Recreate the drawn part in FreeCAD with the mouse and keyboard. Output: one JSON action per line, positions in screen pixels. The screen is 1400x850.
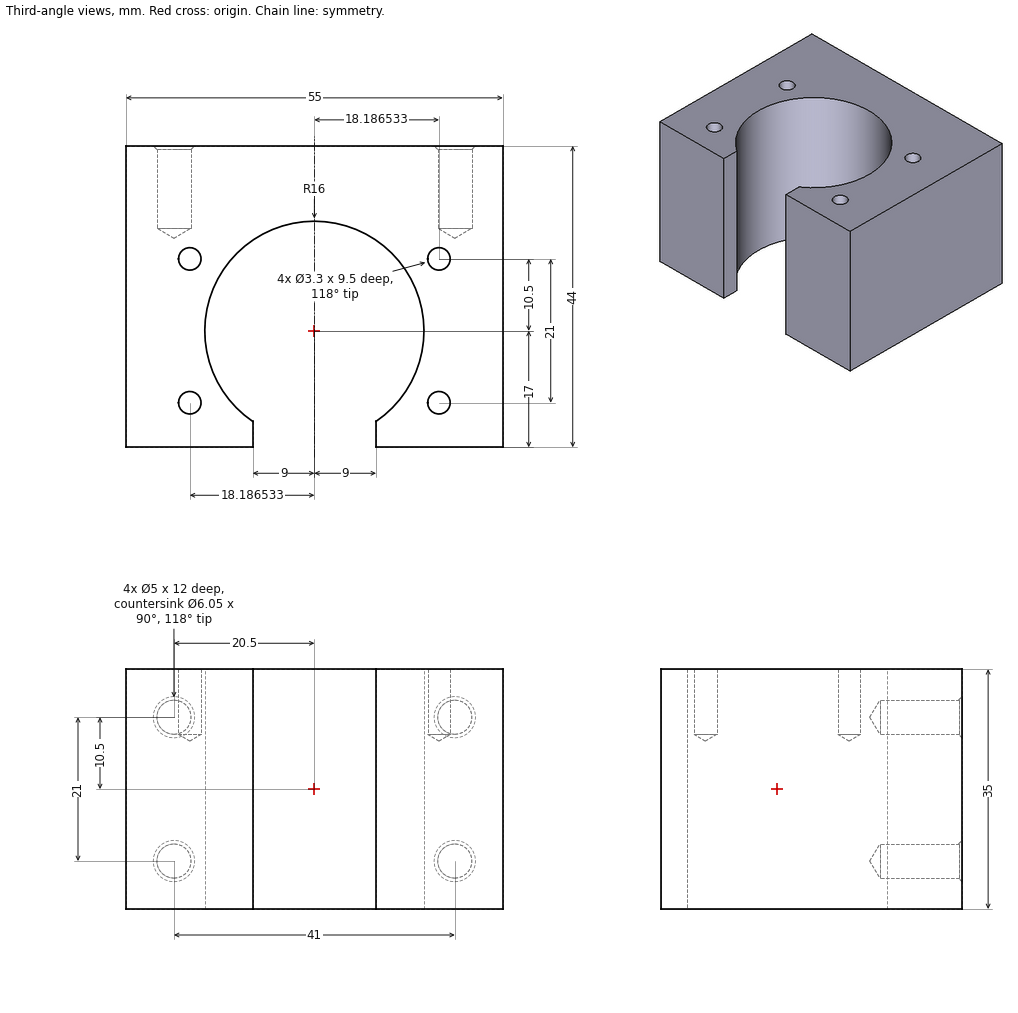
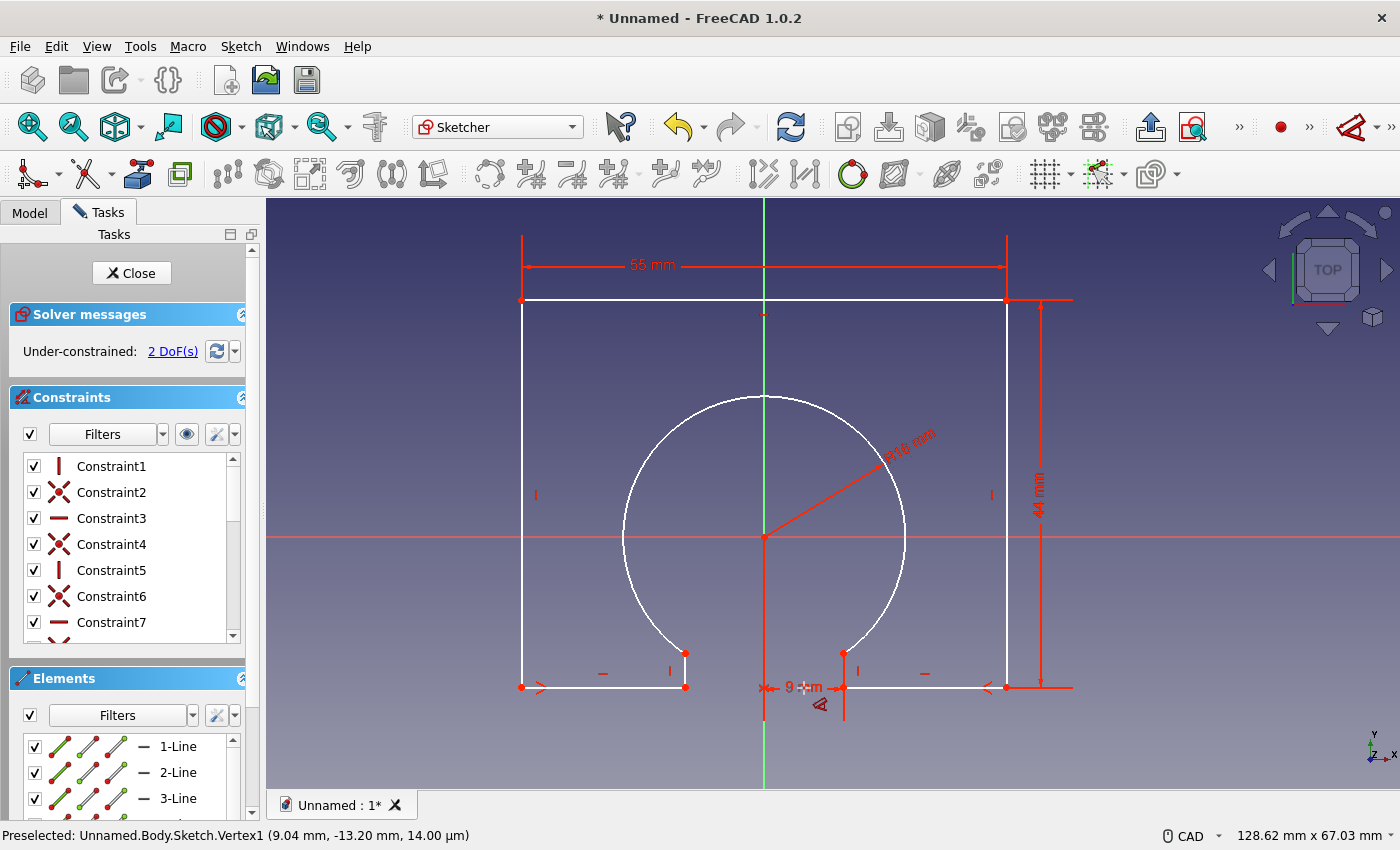
{"action": "left_click", "coordinate": [685, 688]}
{"action": "left_click", "coordinate": [725, 722]}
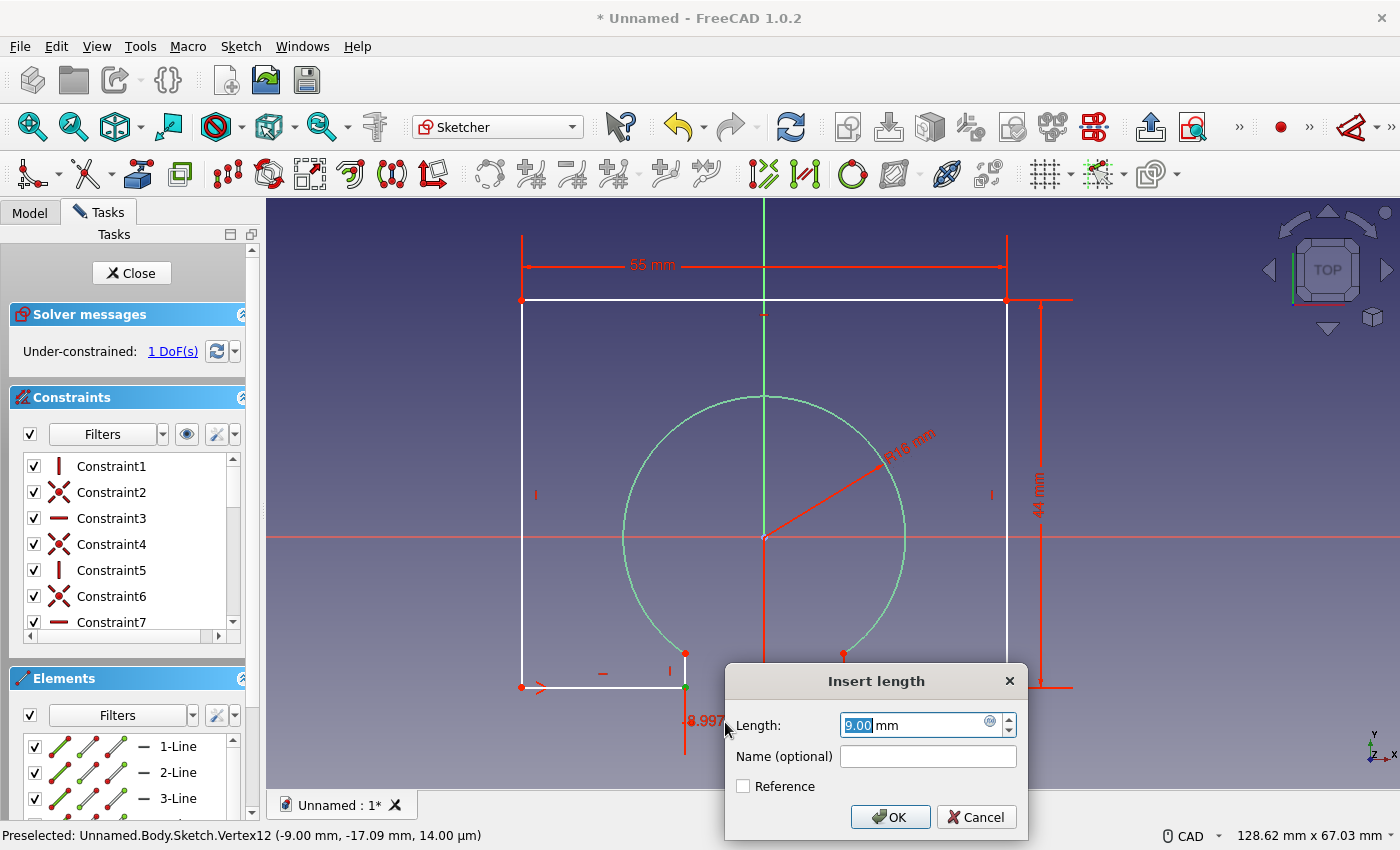
{"action": "type", "text": "9"}
{"action": "key", "text": "Return"}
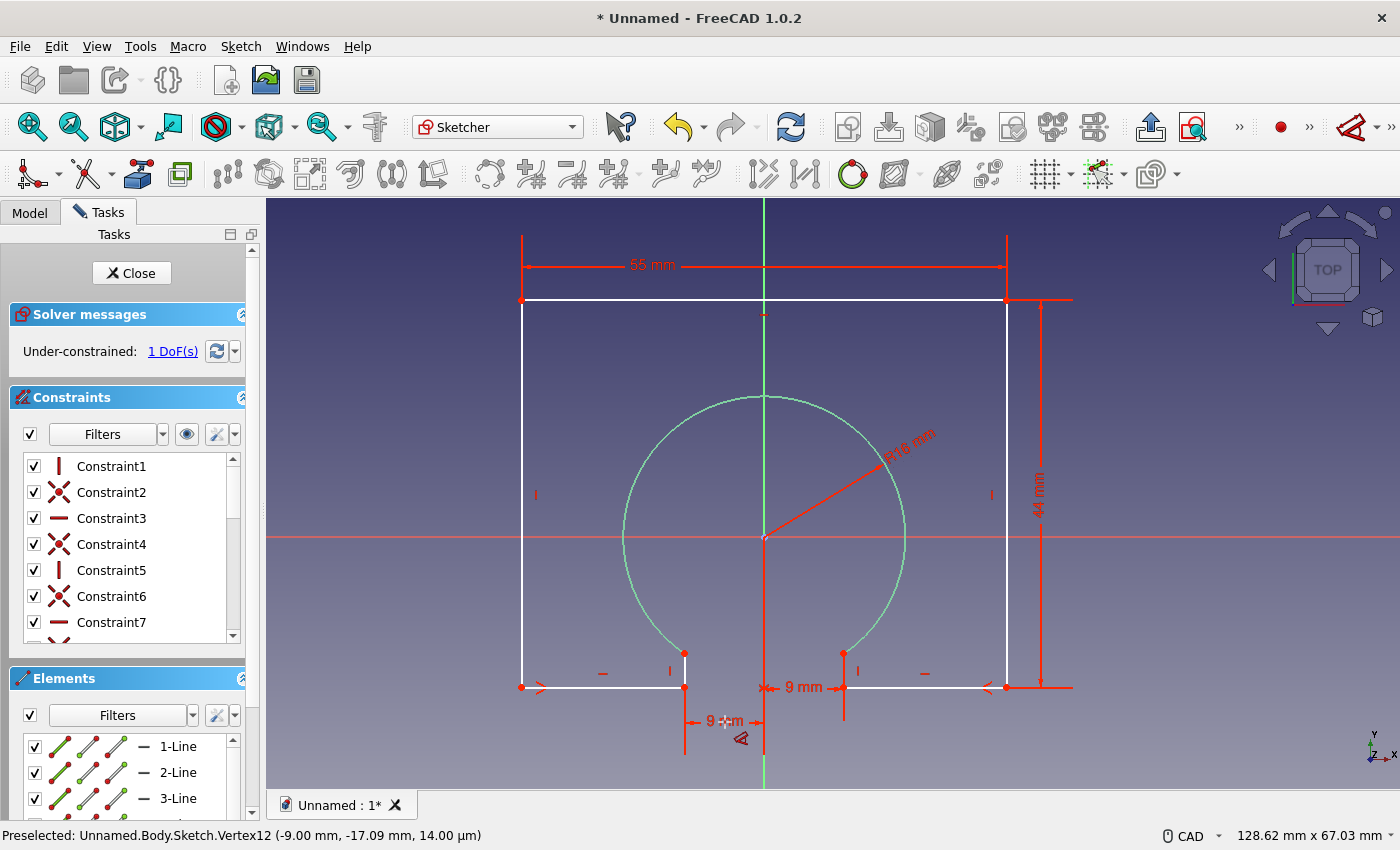
{"action": "left_click", "coordinate": [844, 688]}
{"action": "left_click", "coordinate": [878, 578]}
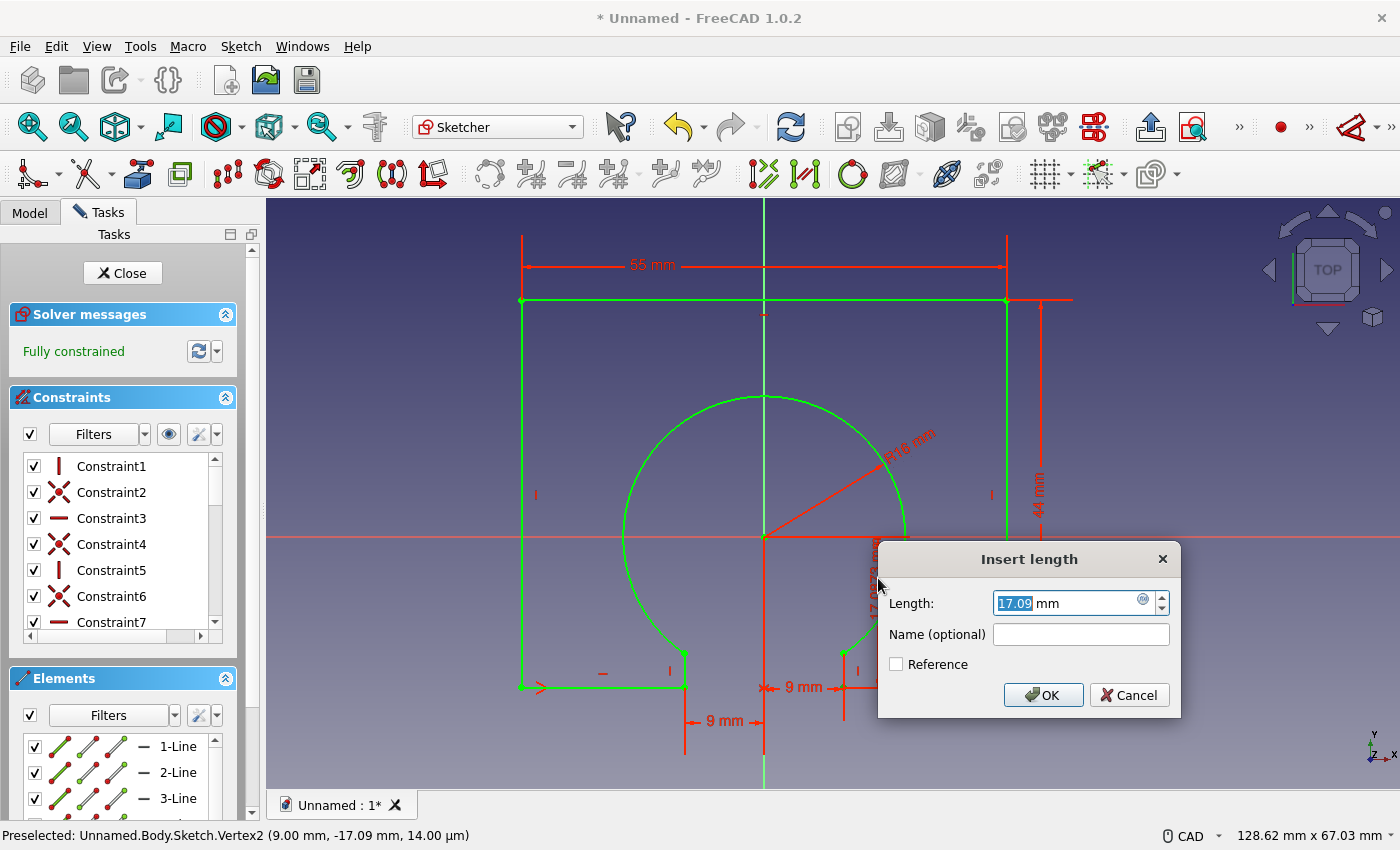
{"action": "type", "text": "17"}
{"action": "key", "text": "Return"}
{"action": "key", "text": "Escape"}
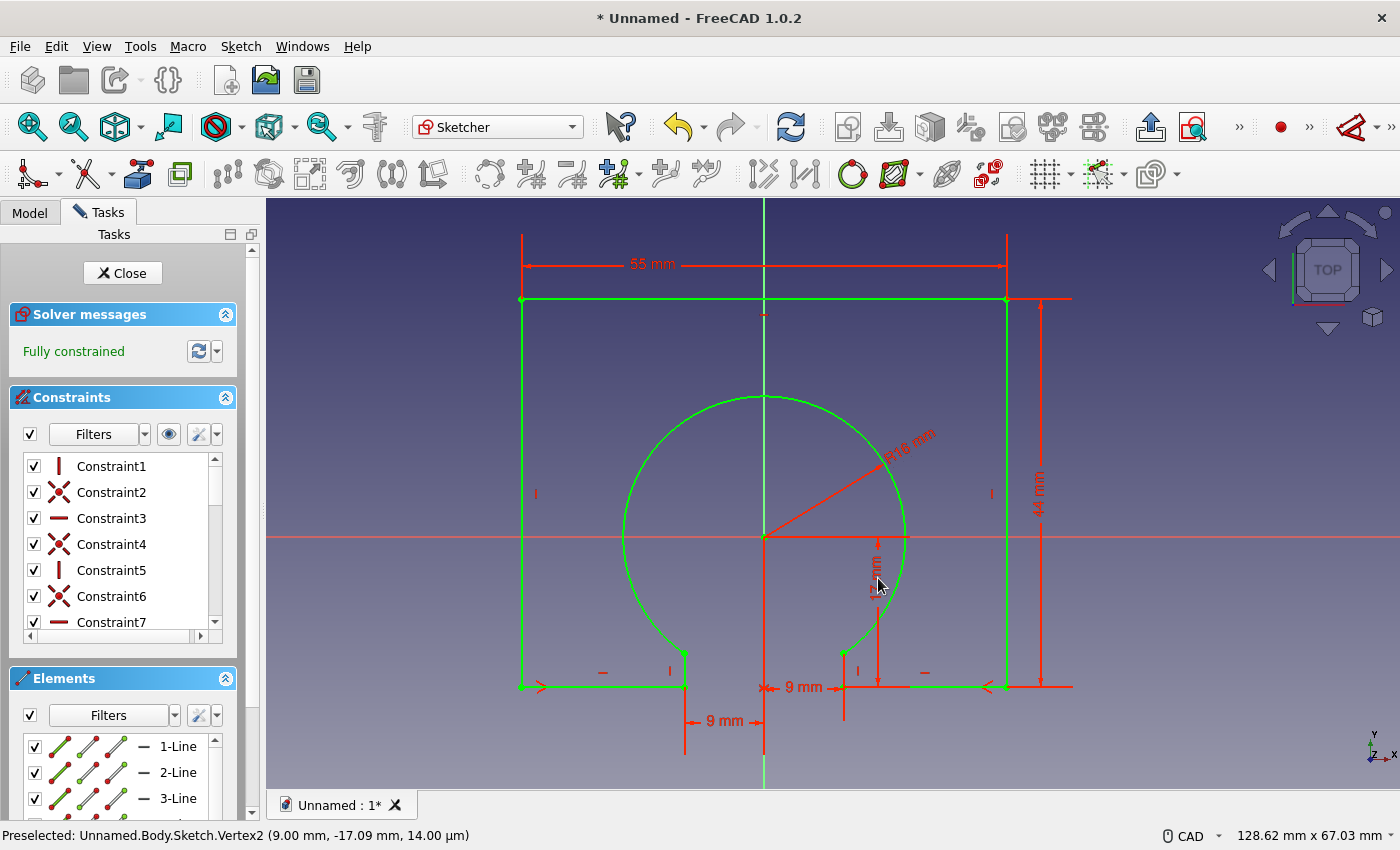
{"action": "left_click", "coordinate": [123, 273]}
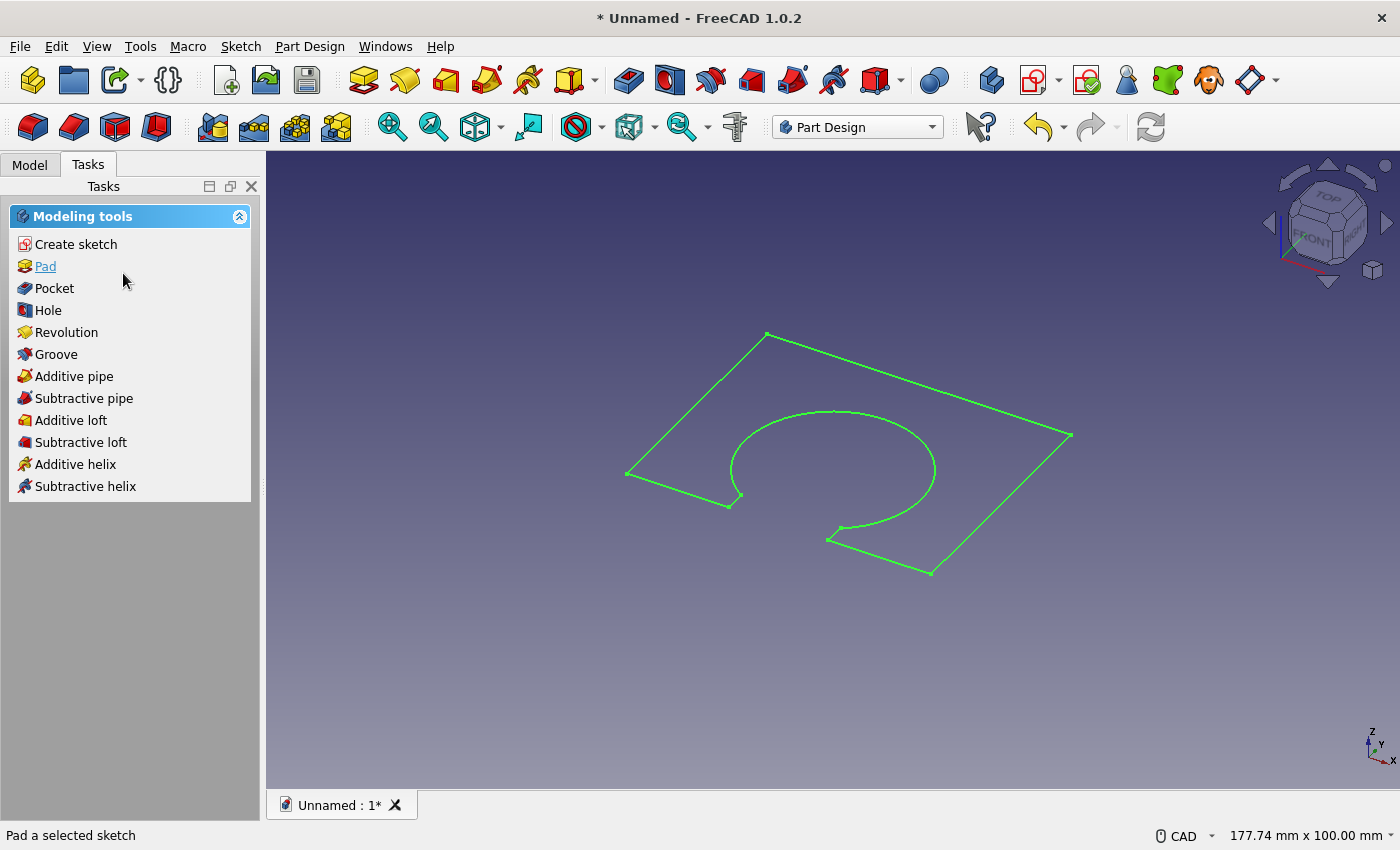
{"action": "left_click", "coordinate": [364, 80]}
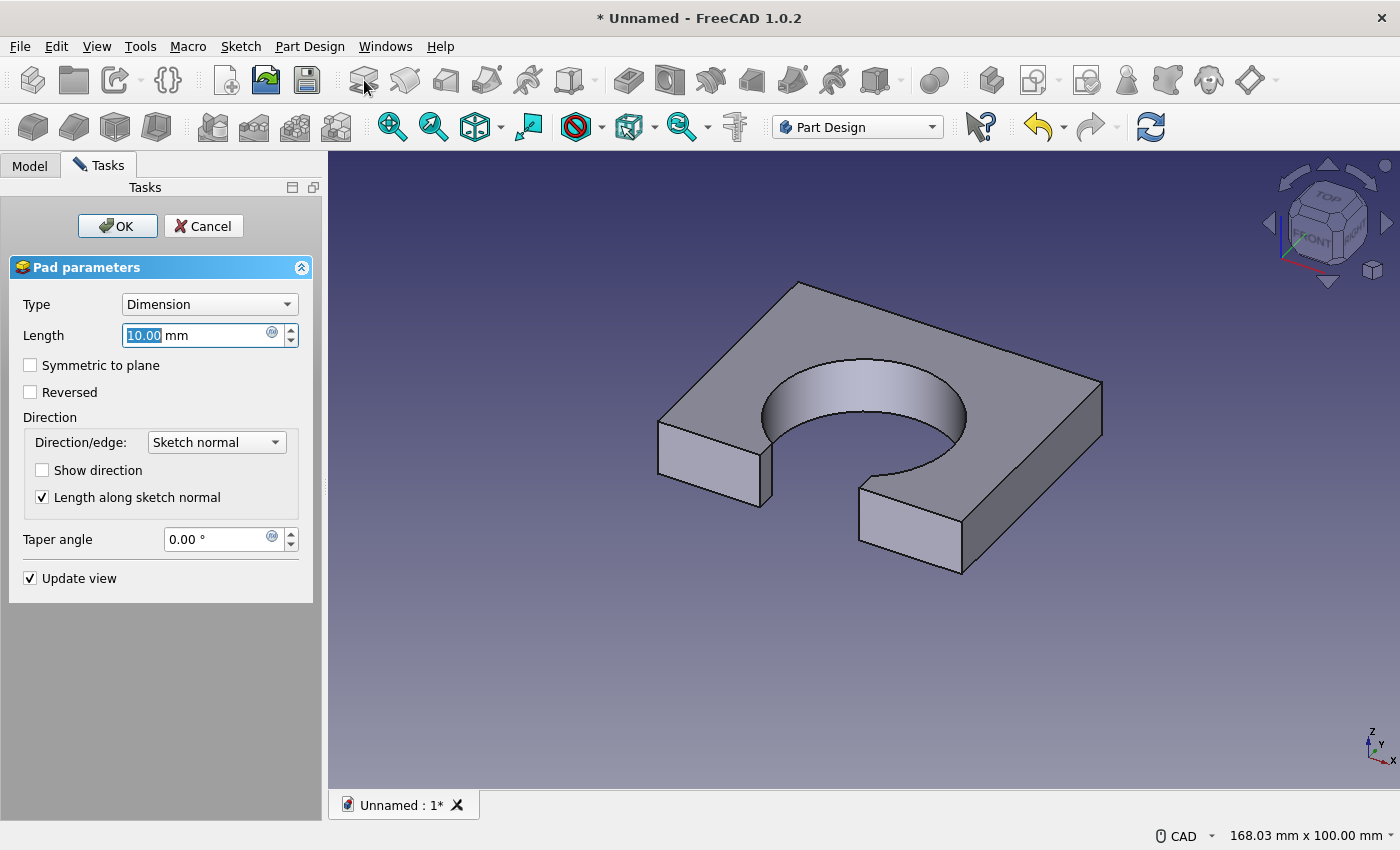
{"action": "type", "text": "35"}
{"action": "key", "text": "Tab"}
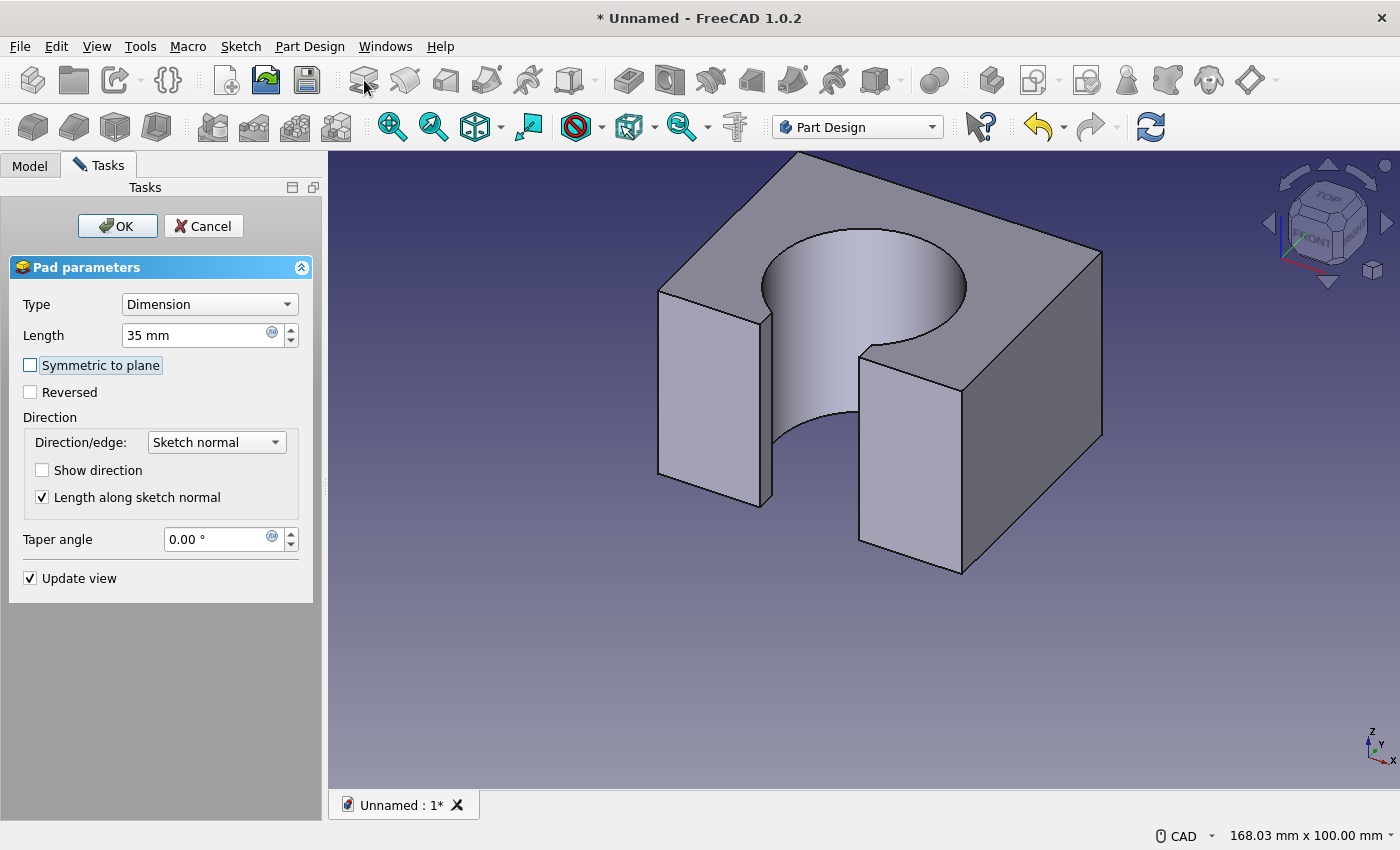
{"action": "left_click", "coordinate": [31, 365]}